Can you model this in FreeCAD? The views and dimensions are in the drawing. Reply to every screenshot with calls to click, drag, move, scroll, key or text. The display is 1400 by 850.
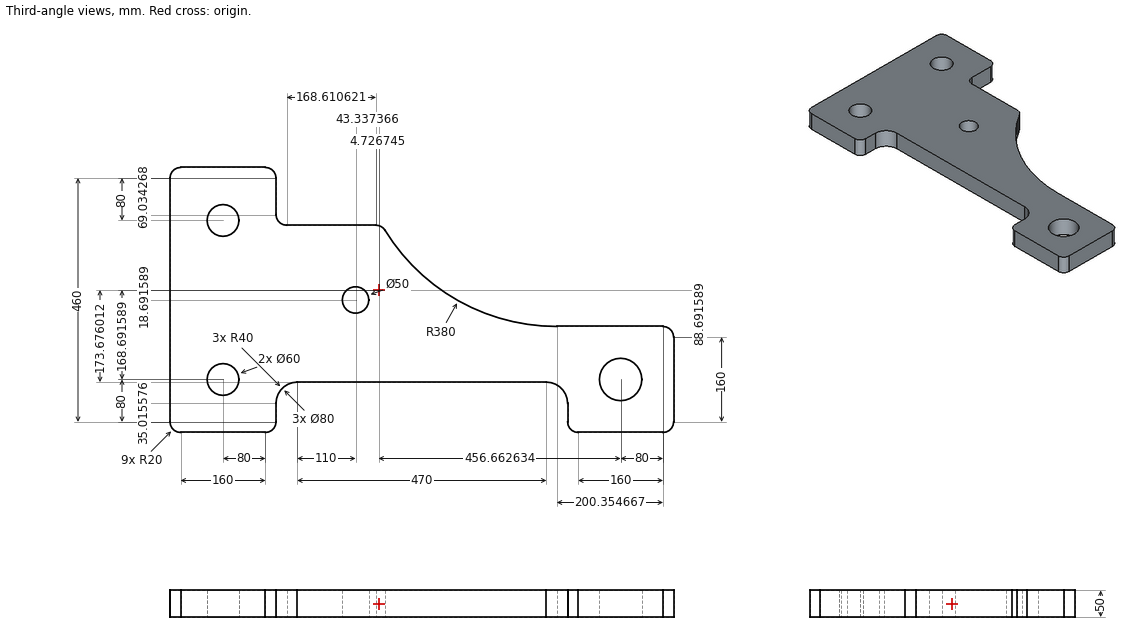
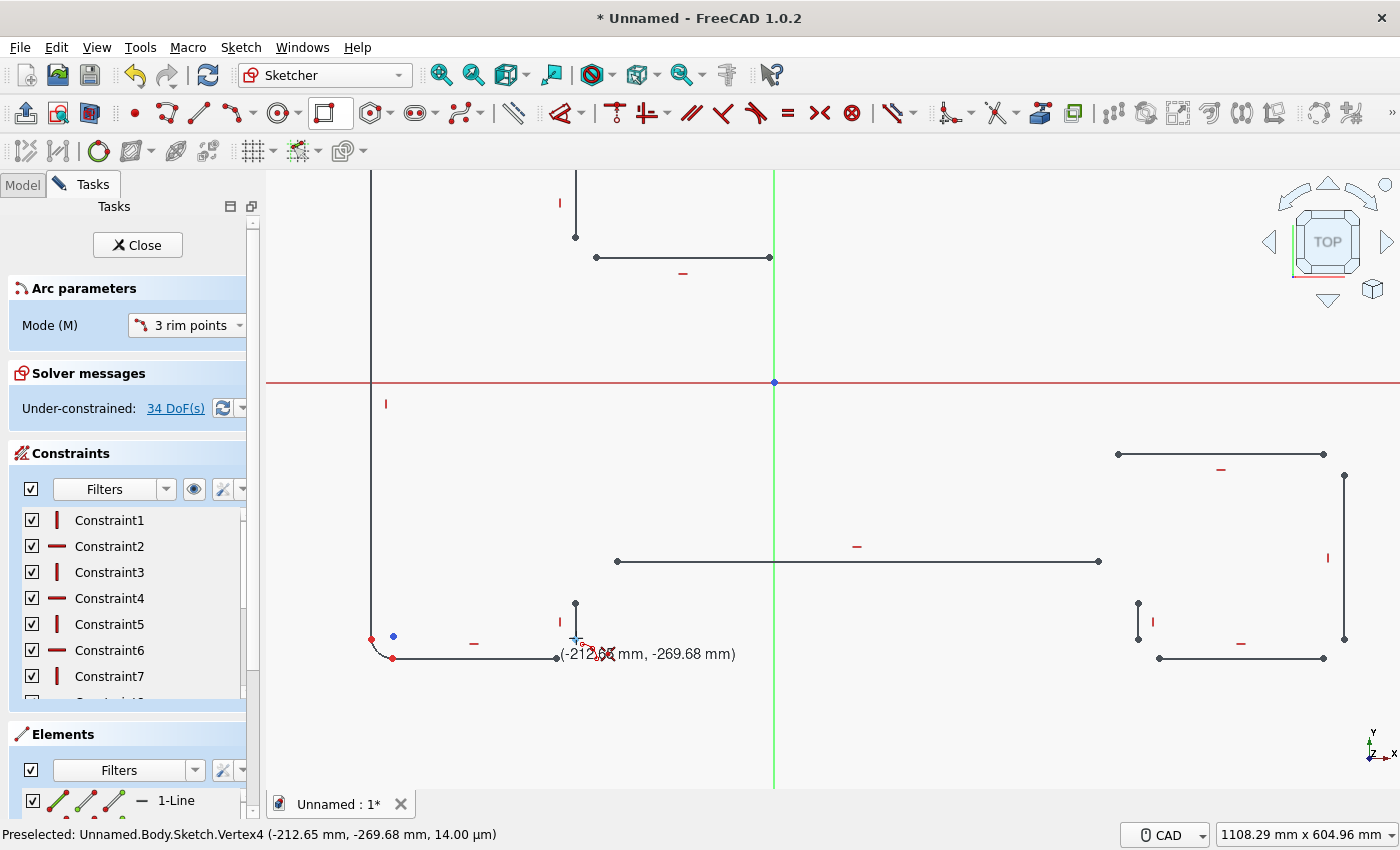
click(576, 639)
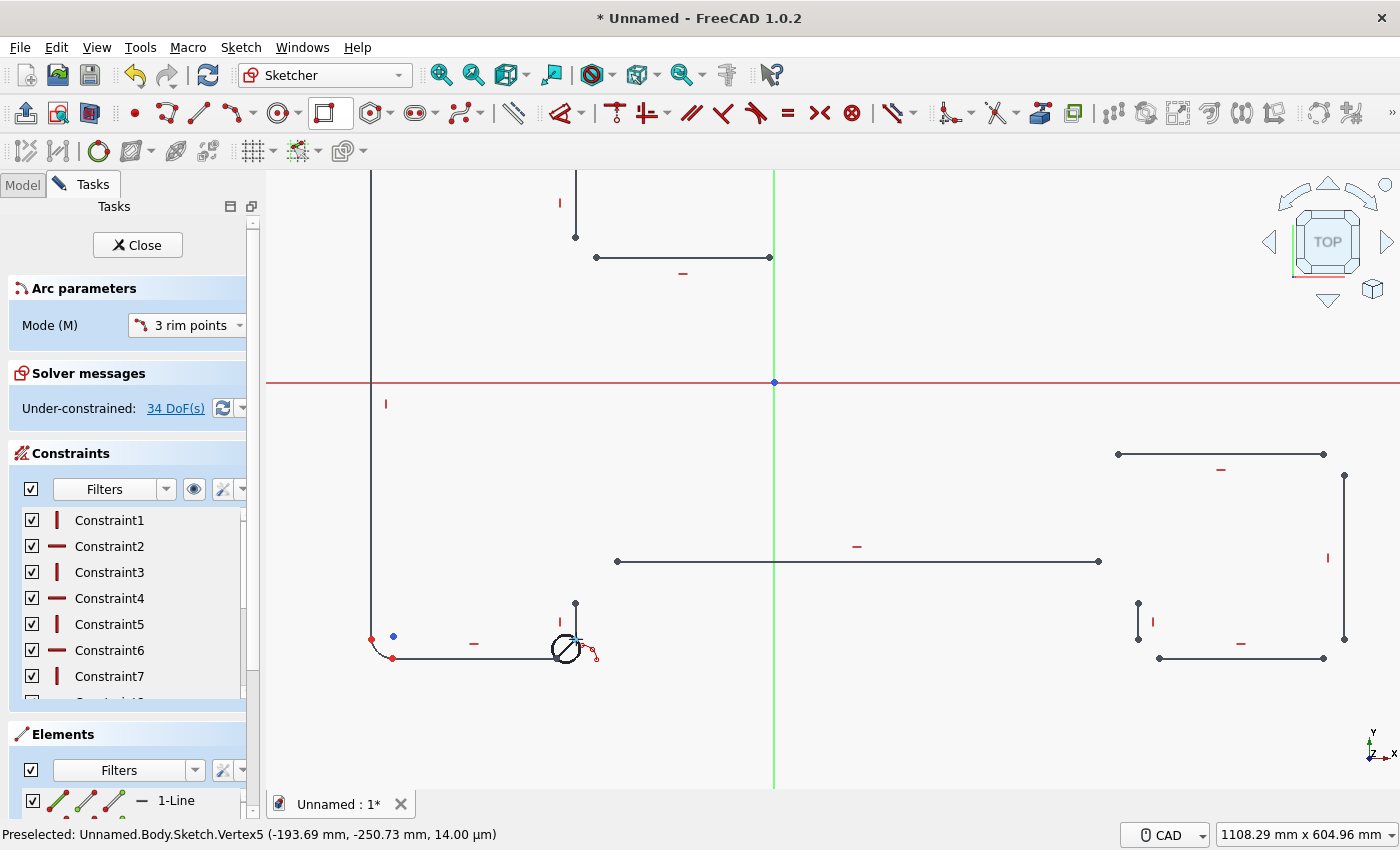
scroll(570, 652, up, 5)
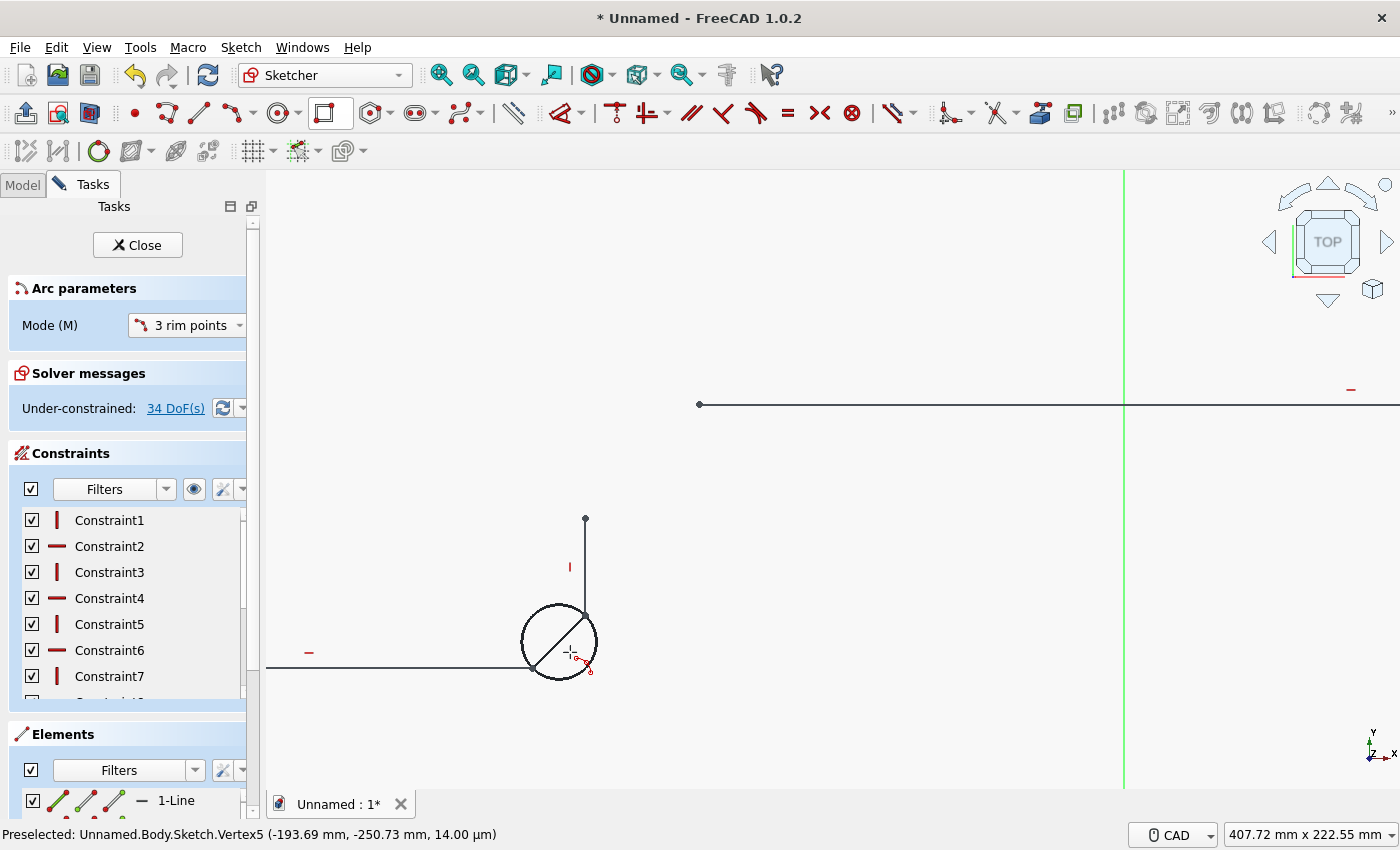
click(570, 649)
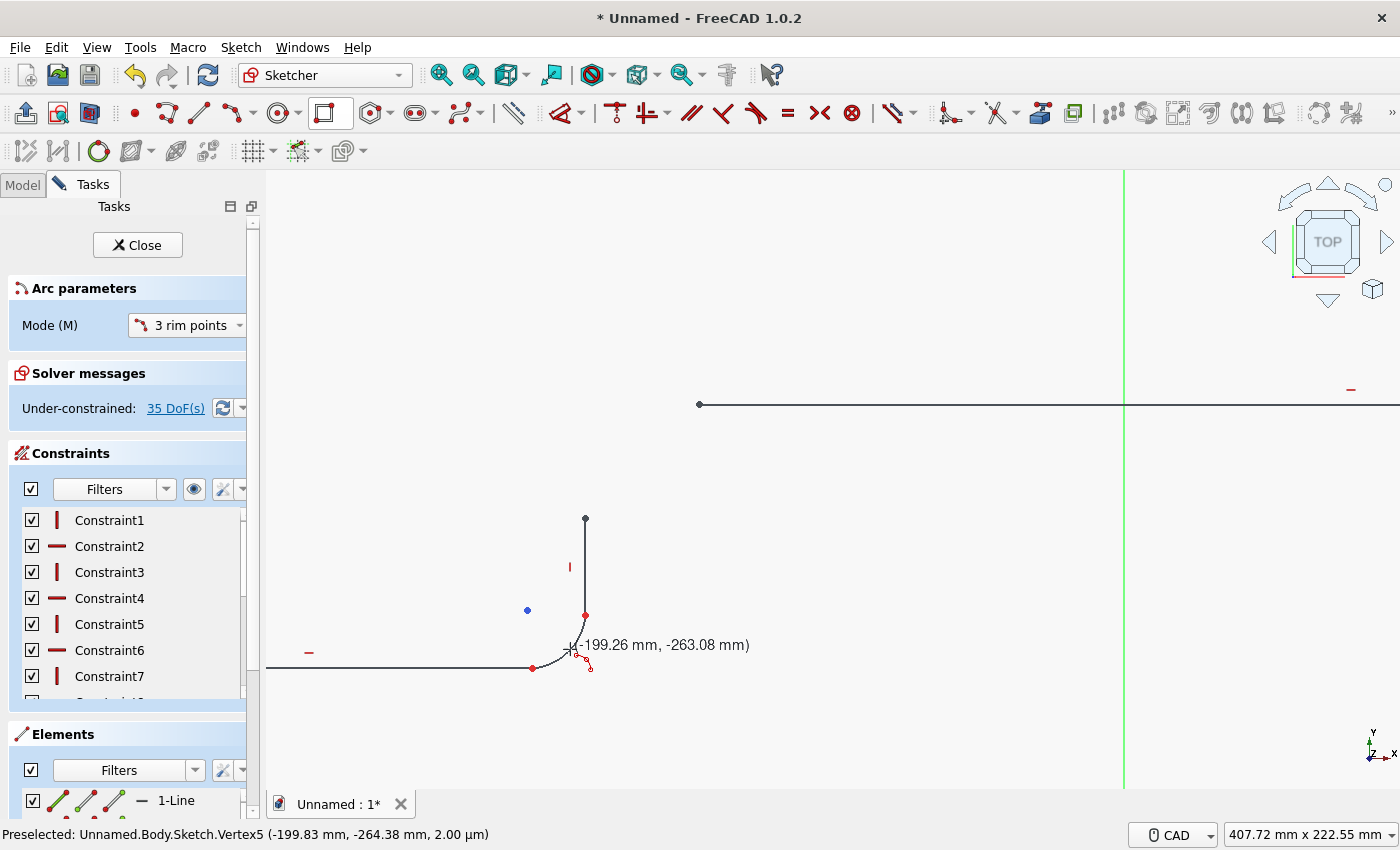
scroll(572, 646, down, 7)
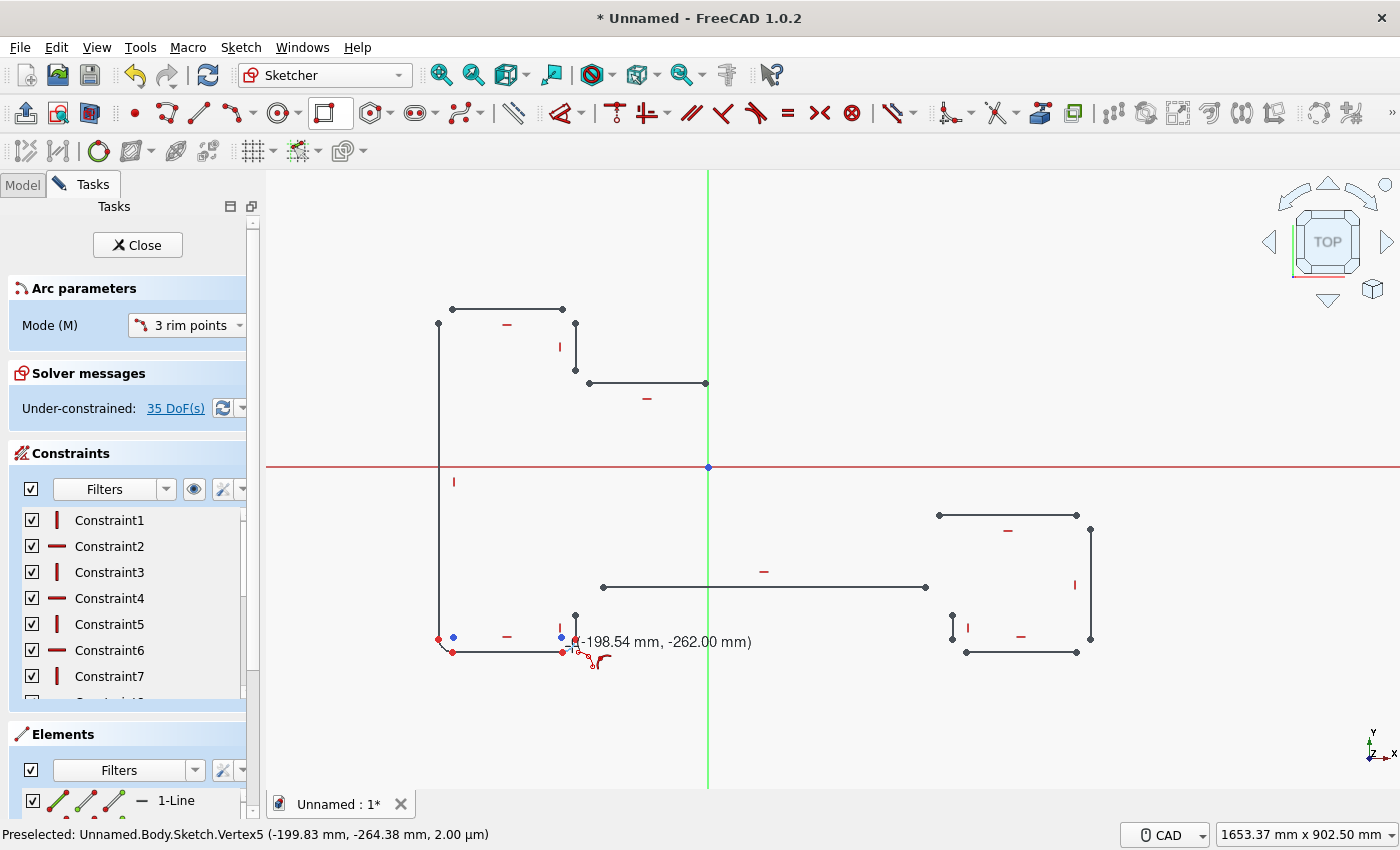
scroll(576, 614, up, 2)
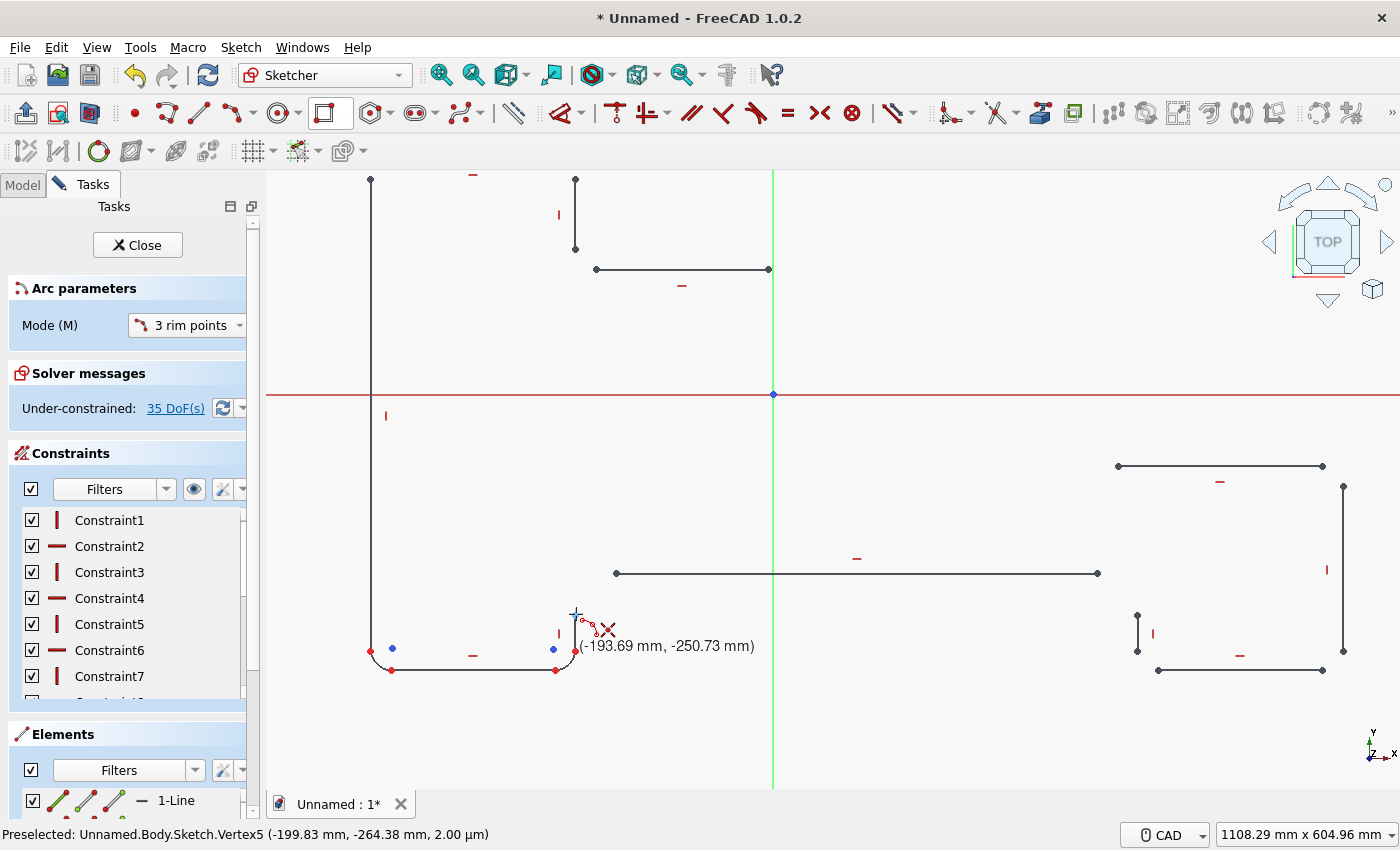
click(575, 615)
click(617, 574)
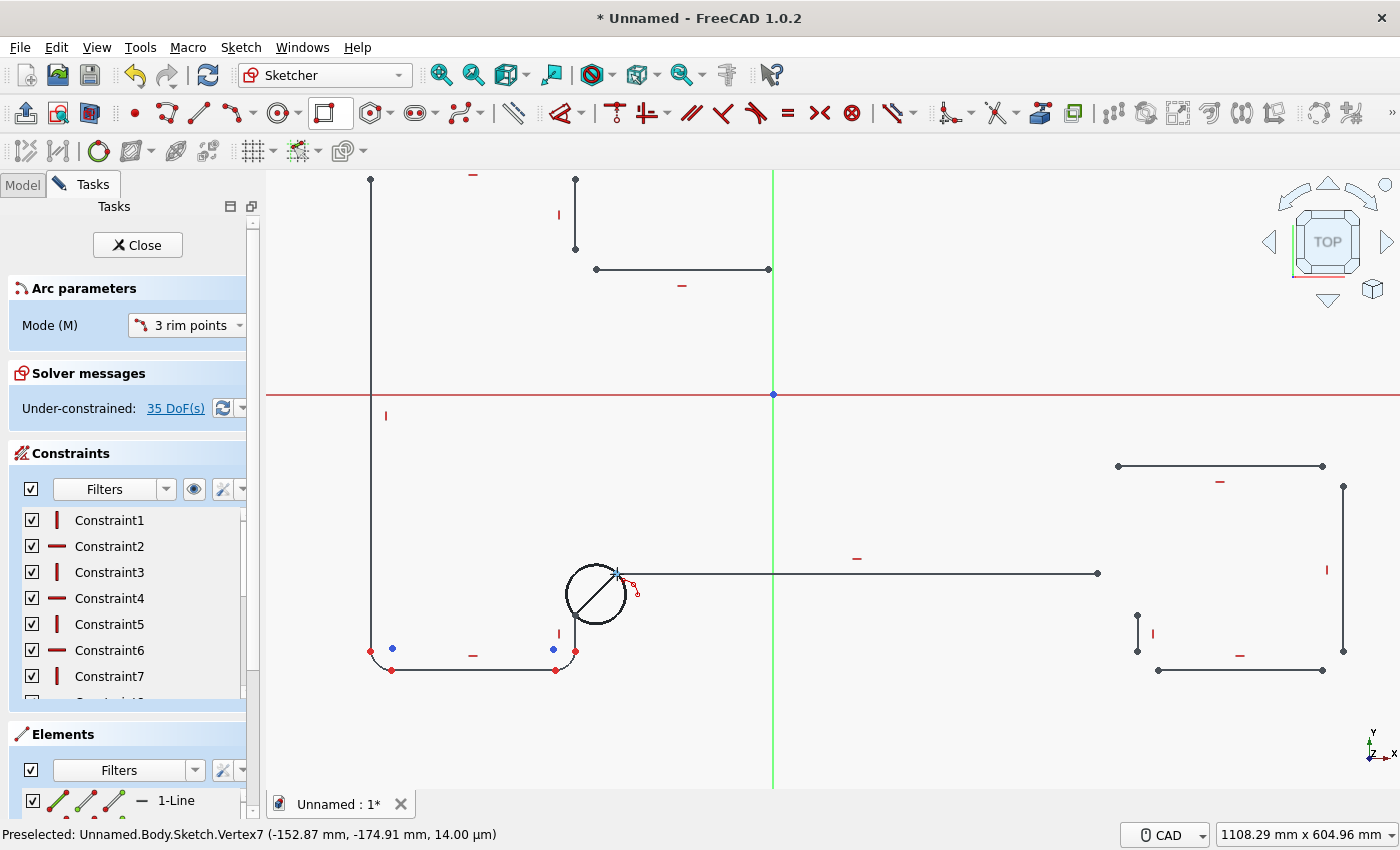
scroll(588, 584, up, 2)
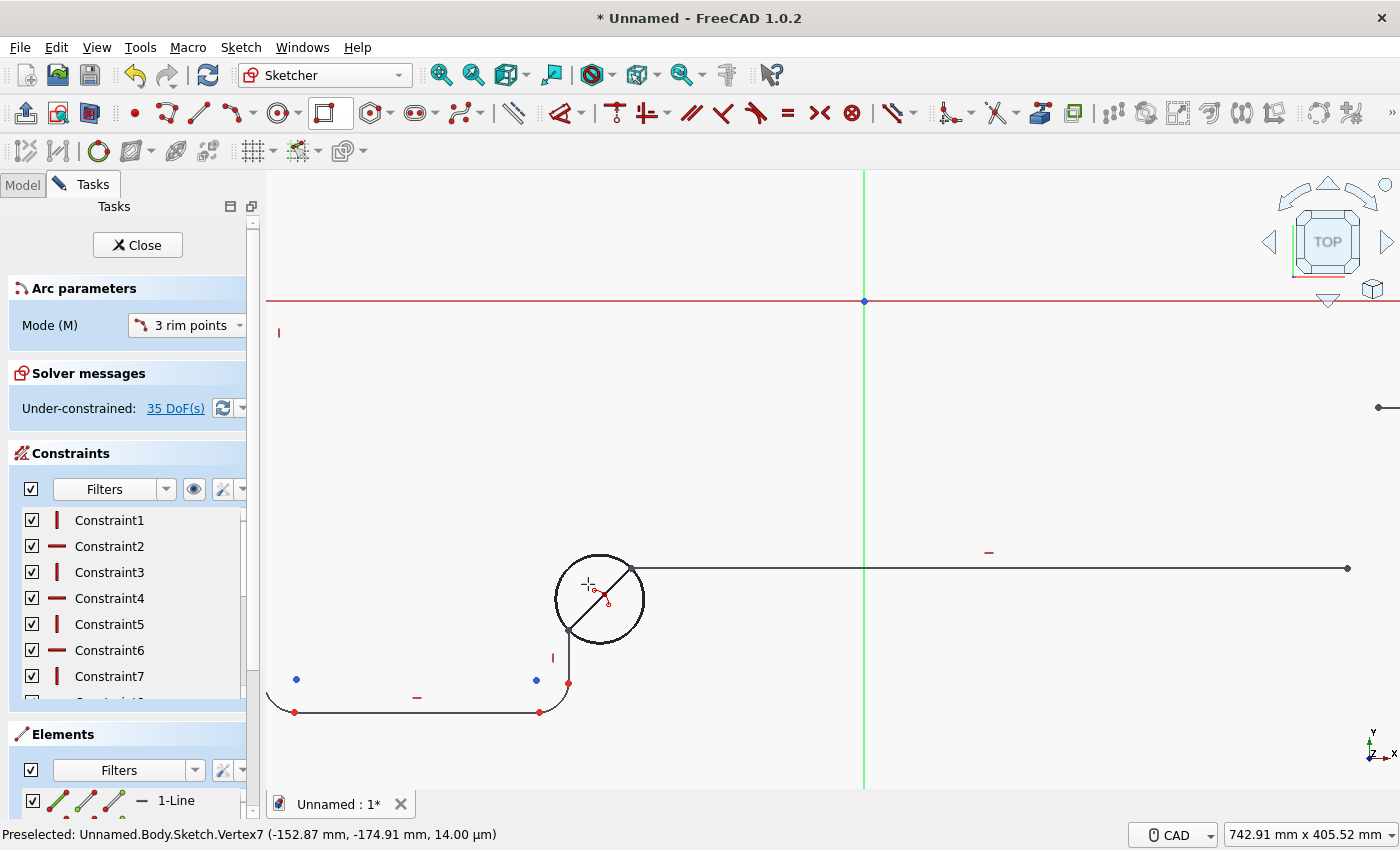
click(587, 584)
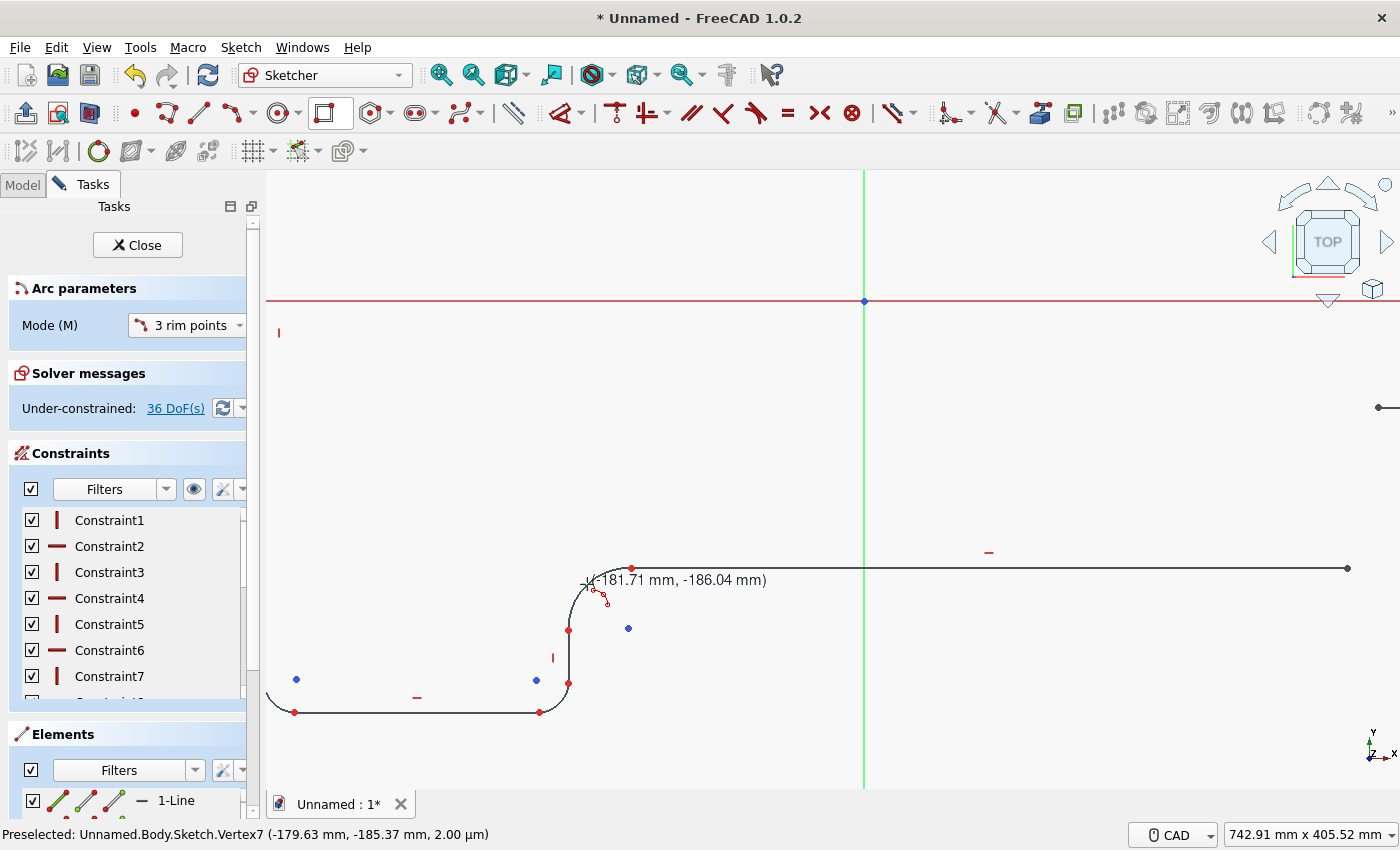
scroll(581, 602, down, 4)